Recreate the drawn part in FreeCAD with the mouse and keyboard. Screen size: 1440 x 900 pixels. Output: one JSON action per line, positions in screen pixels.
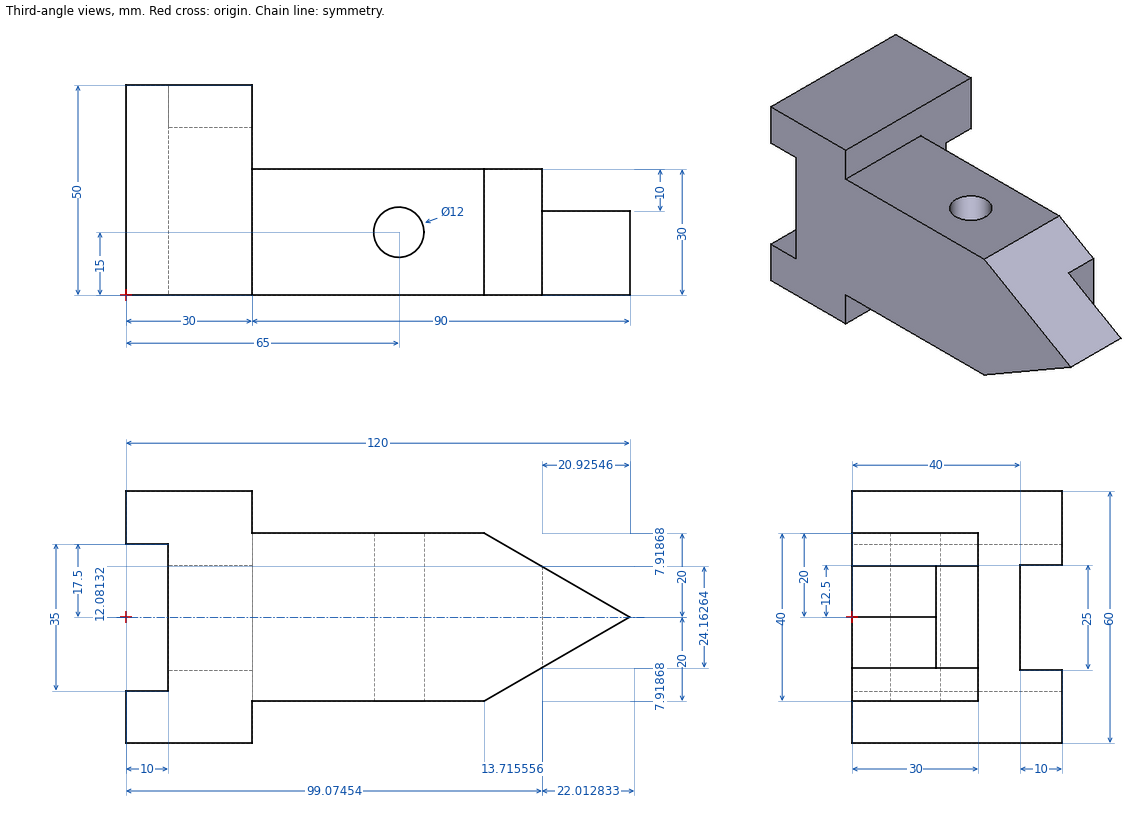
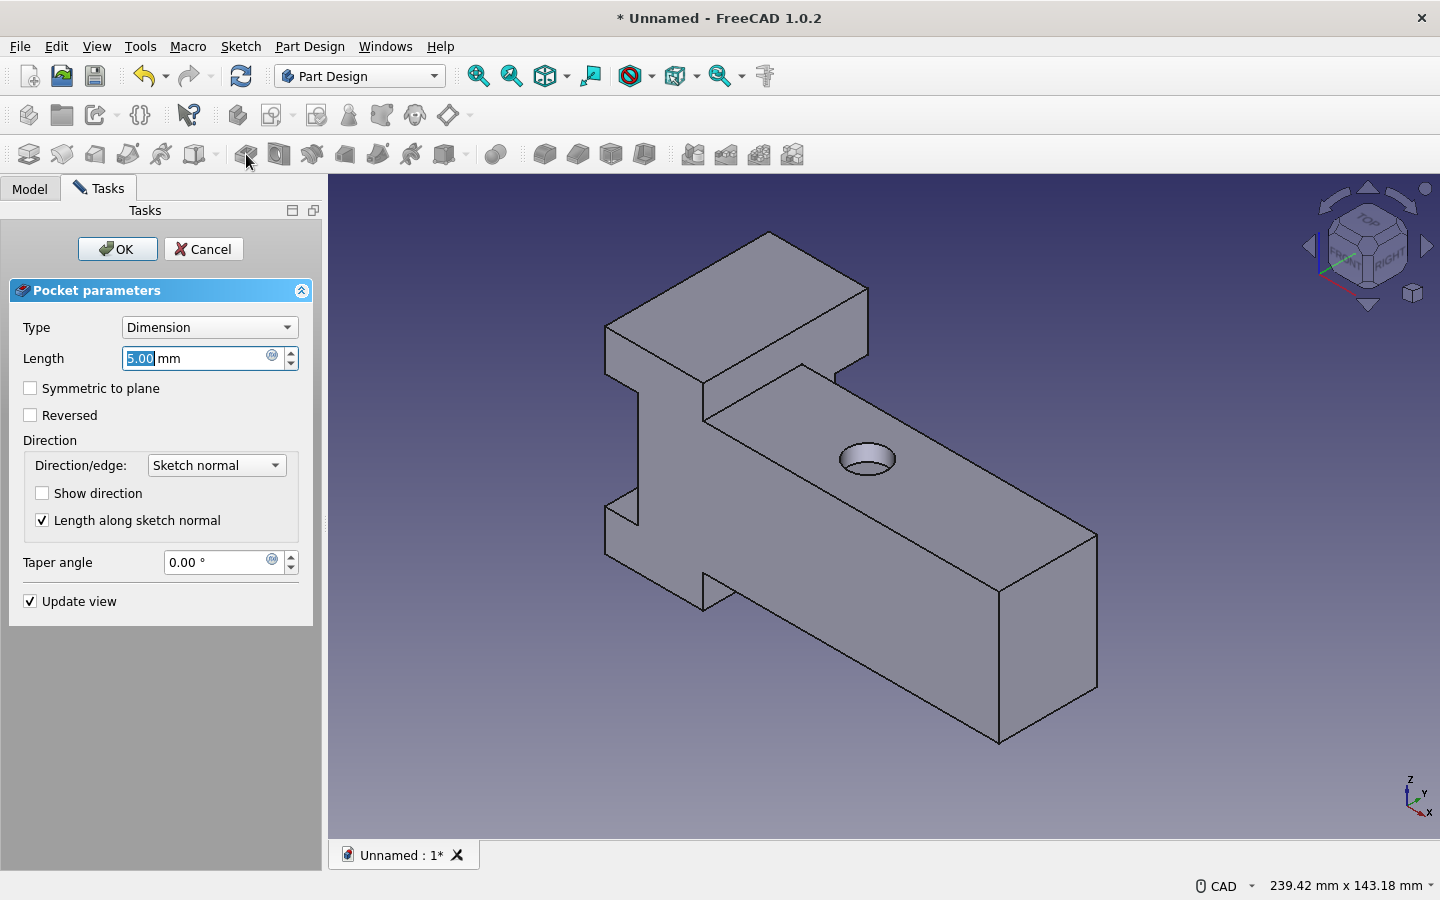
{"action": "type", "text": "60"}
{"action": "key", "text": "Tab"}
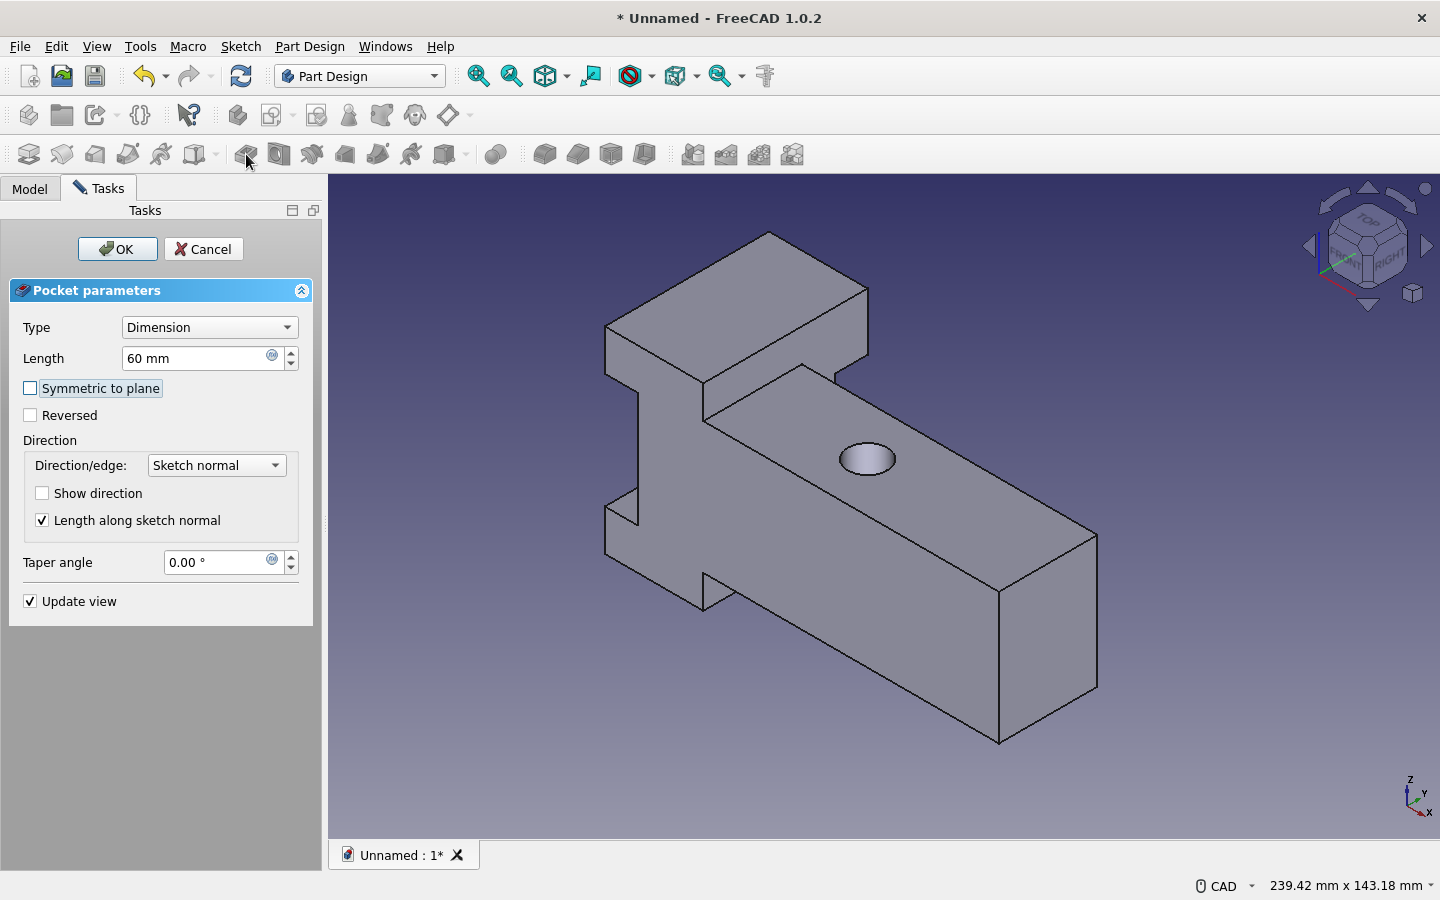
{"action": "left_click", "coordinate": [118, 249]}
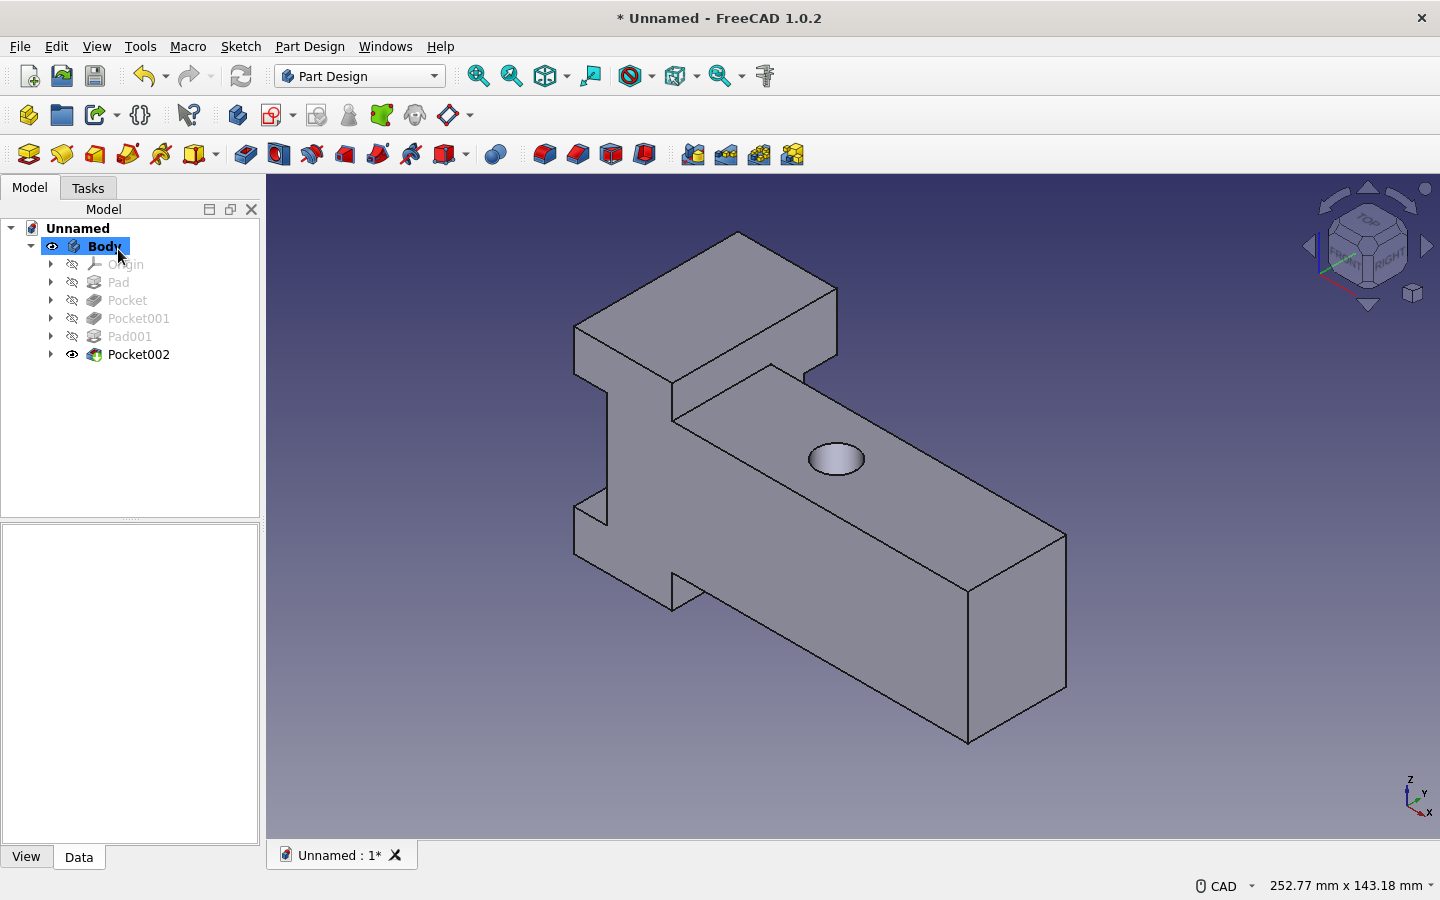
{"action": "key", "text": "4"}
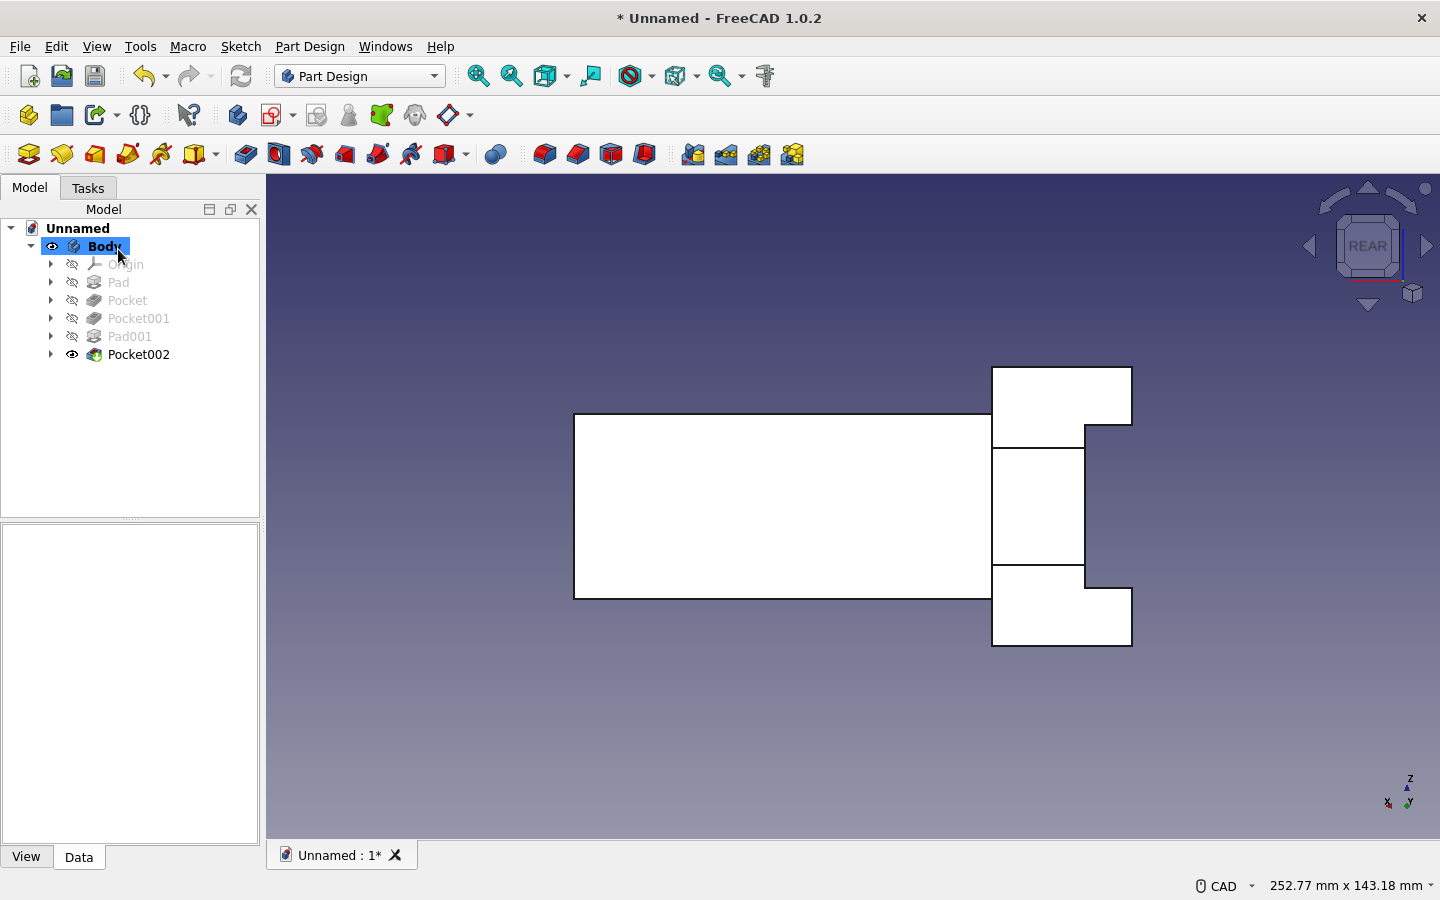
{"action": "left_click", "coordinate": [724, 506]}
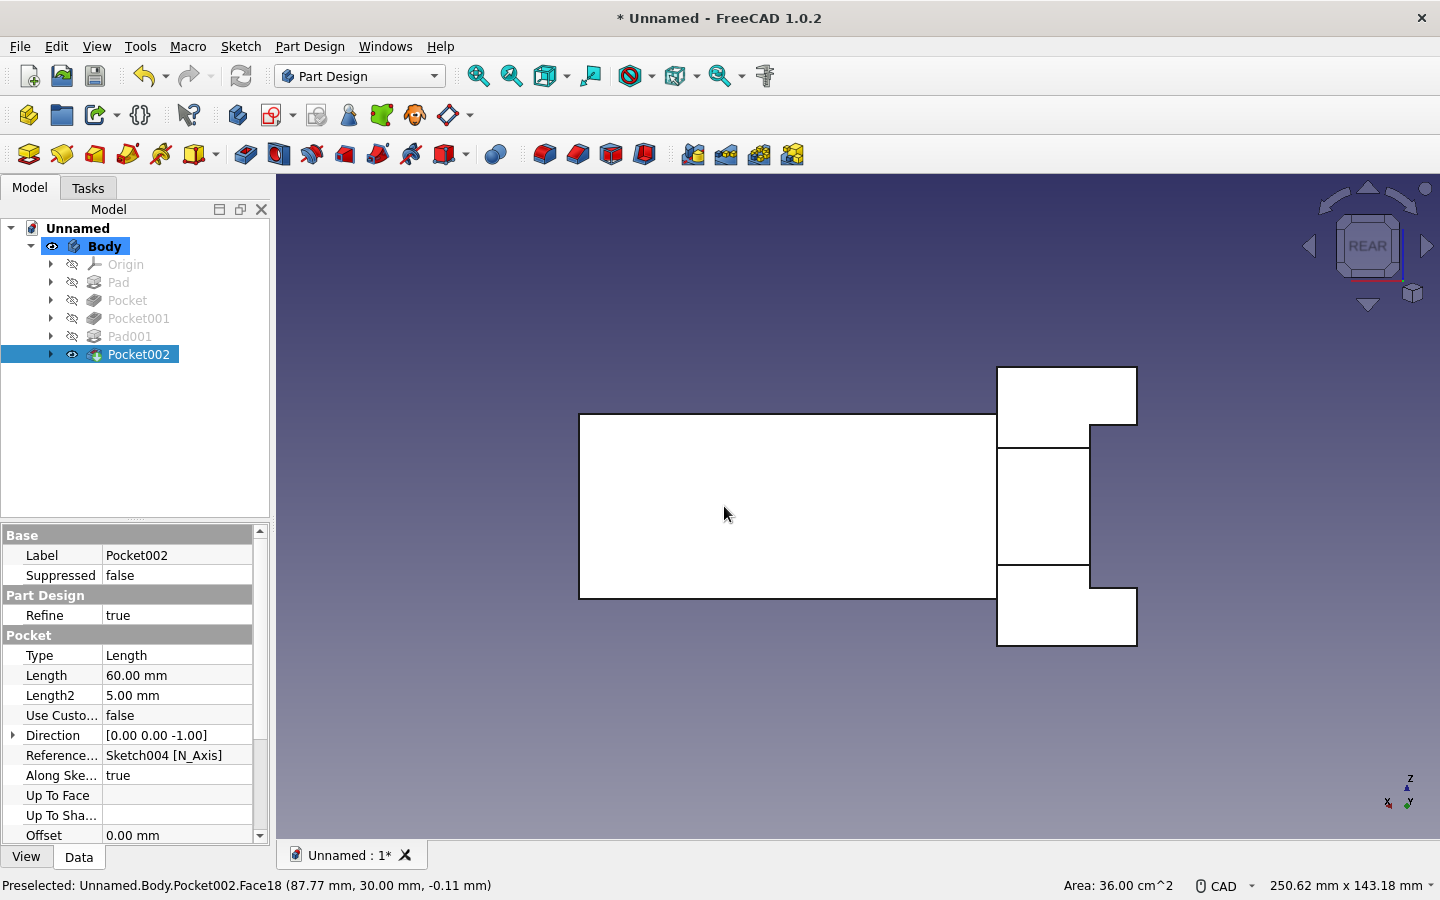
{"action": "left_click", "coordinate": [270, 116]}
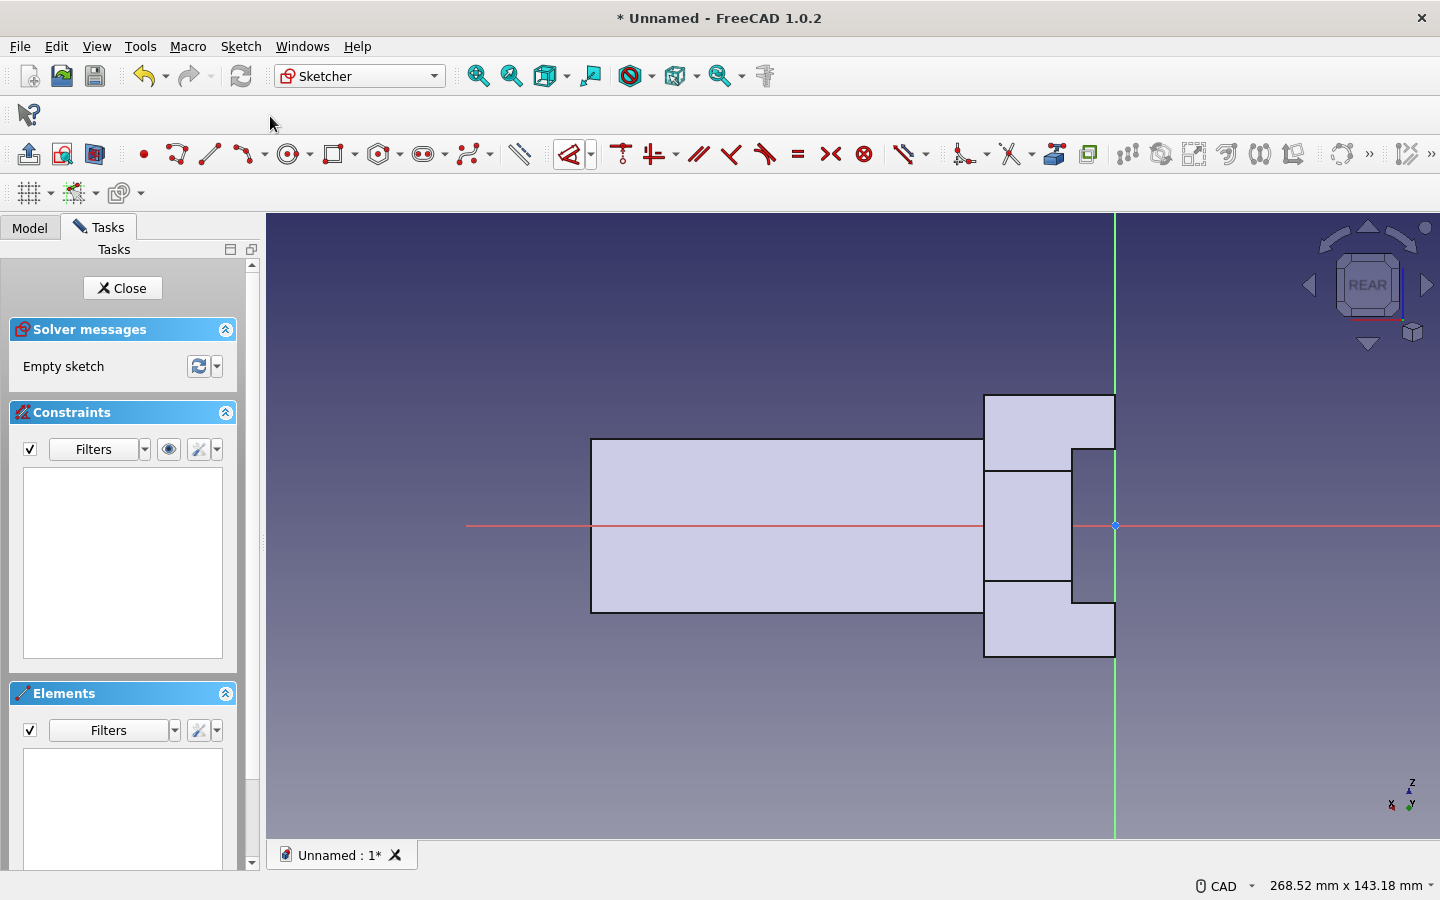
{"action": "key", "text": "q s"}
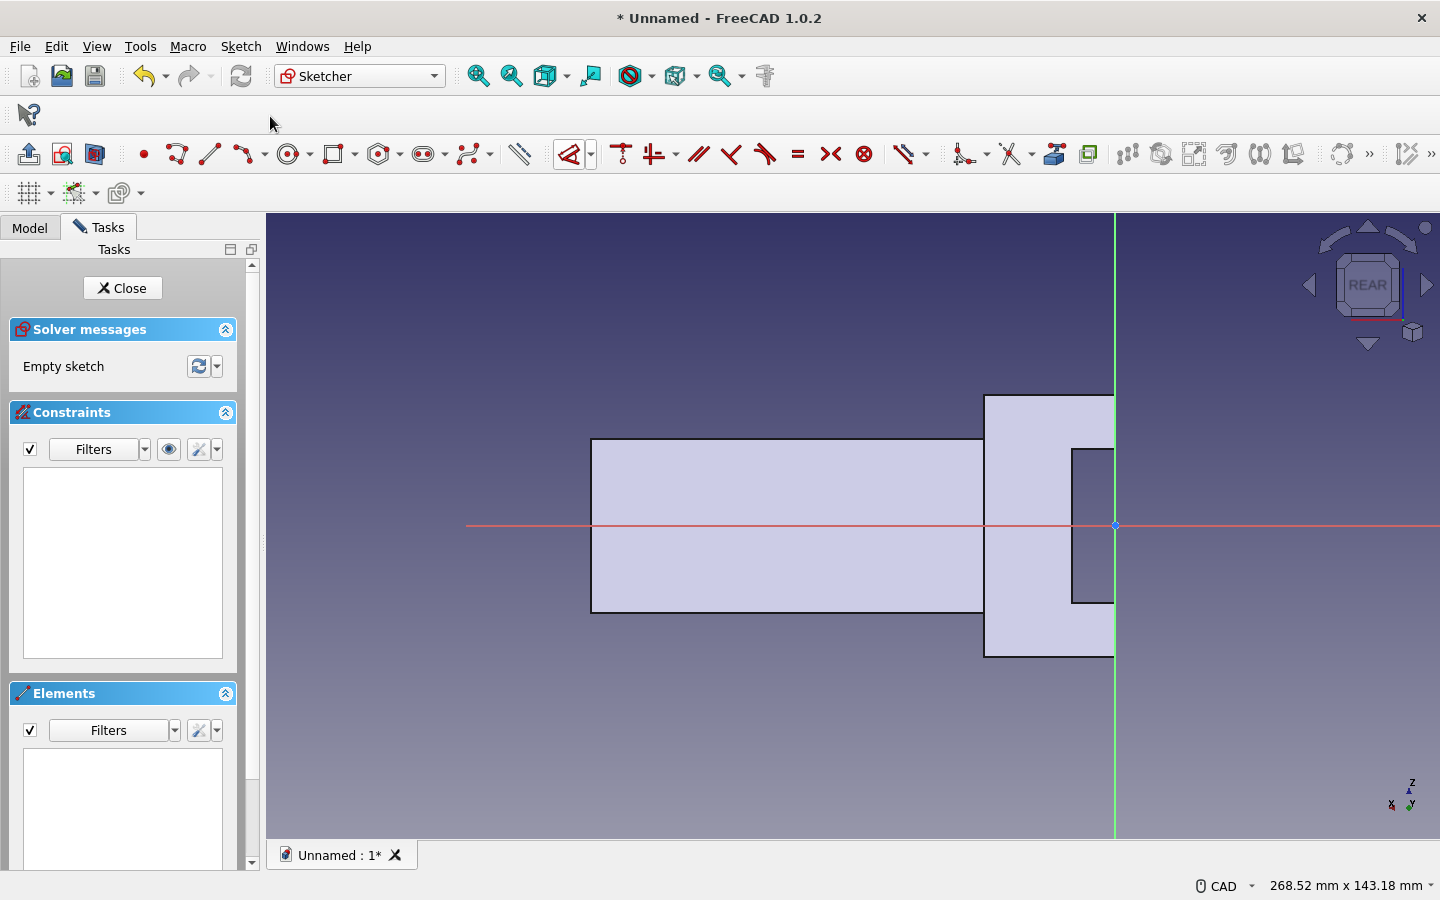
{"action": "scroll", "coordinate": [516, 526], "scroll_direction": "up", "scroll_amount": 4}